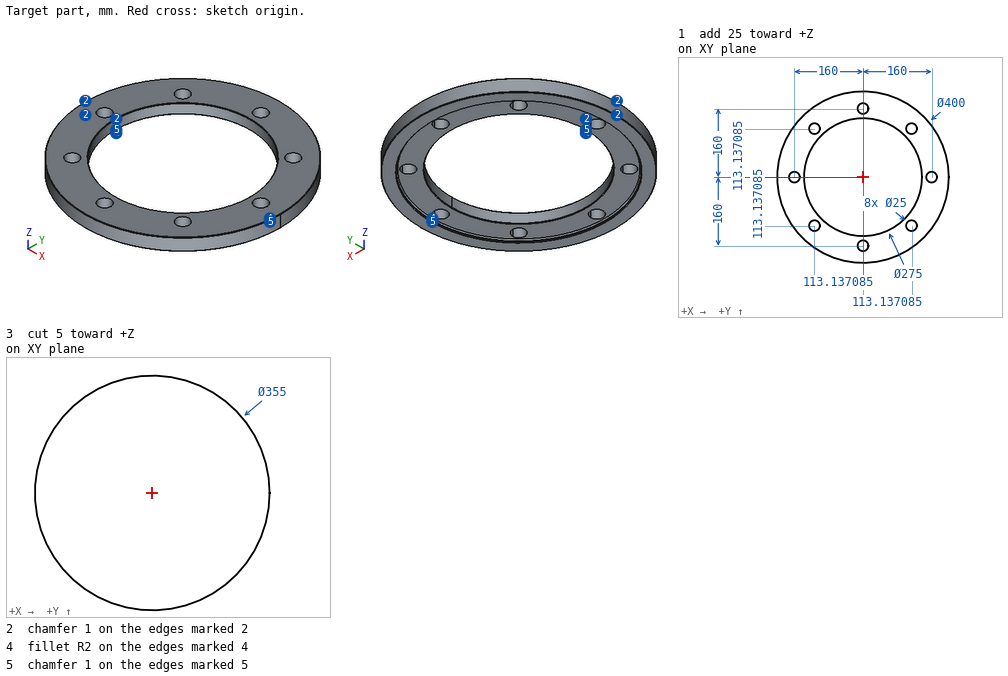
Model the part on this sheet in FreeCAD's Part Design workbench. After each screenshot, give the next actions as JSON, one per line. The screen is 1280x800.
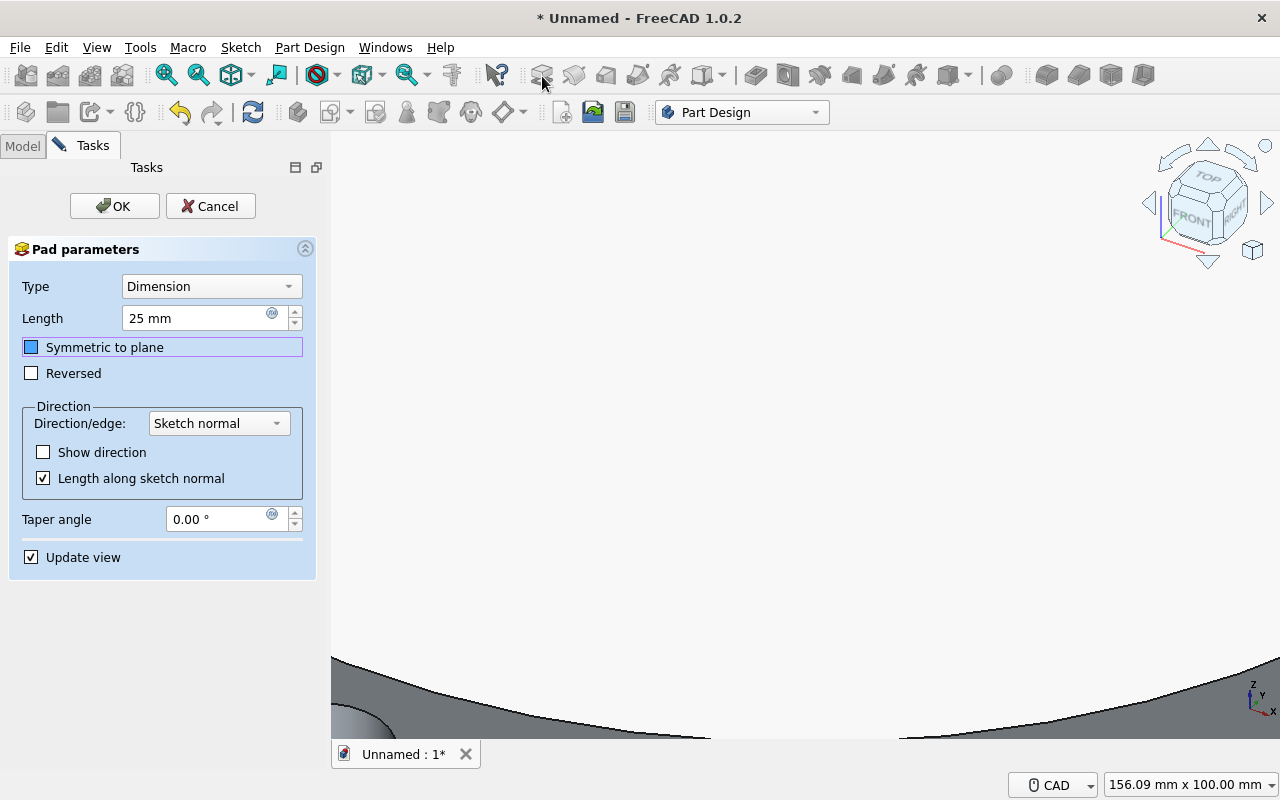
{"action": "left_click", "coordinate": [115, 206]}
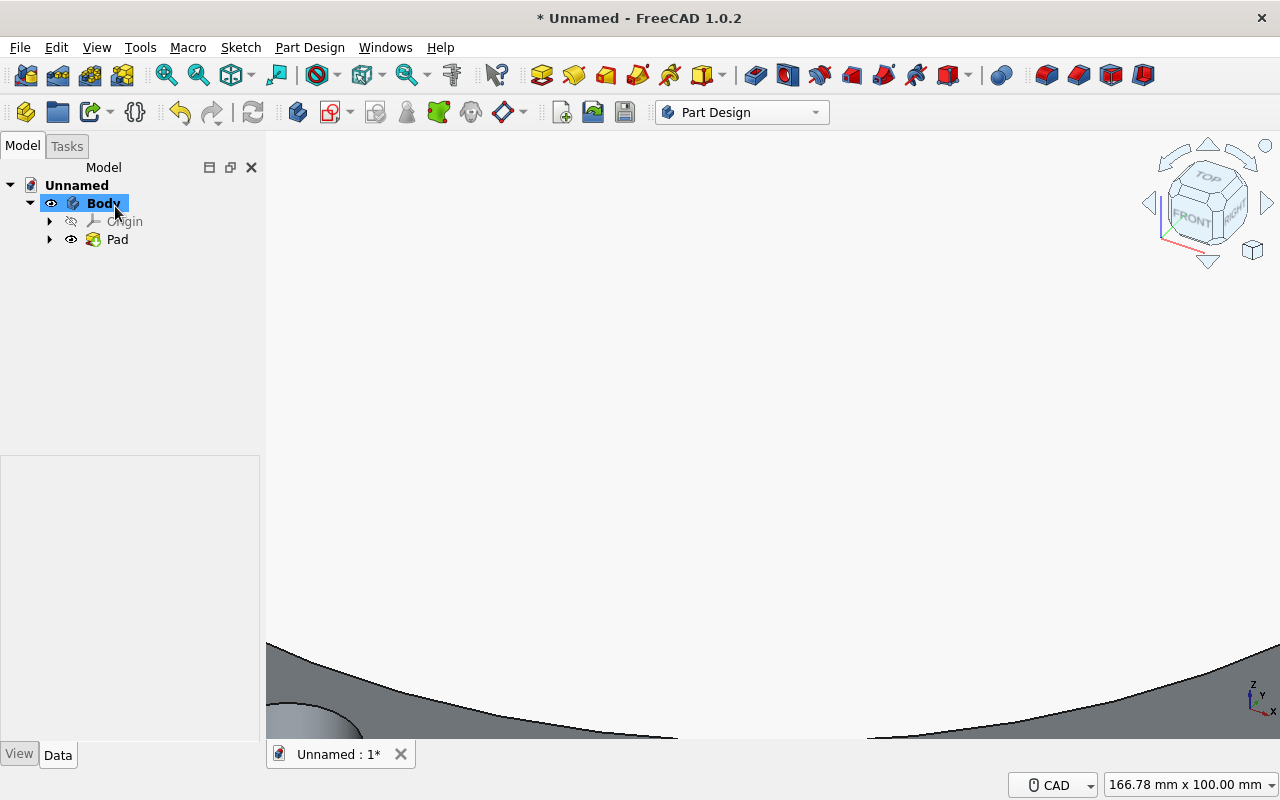
{"action": "left_click", "coordinate": [168, 76]}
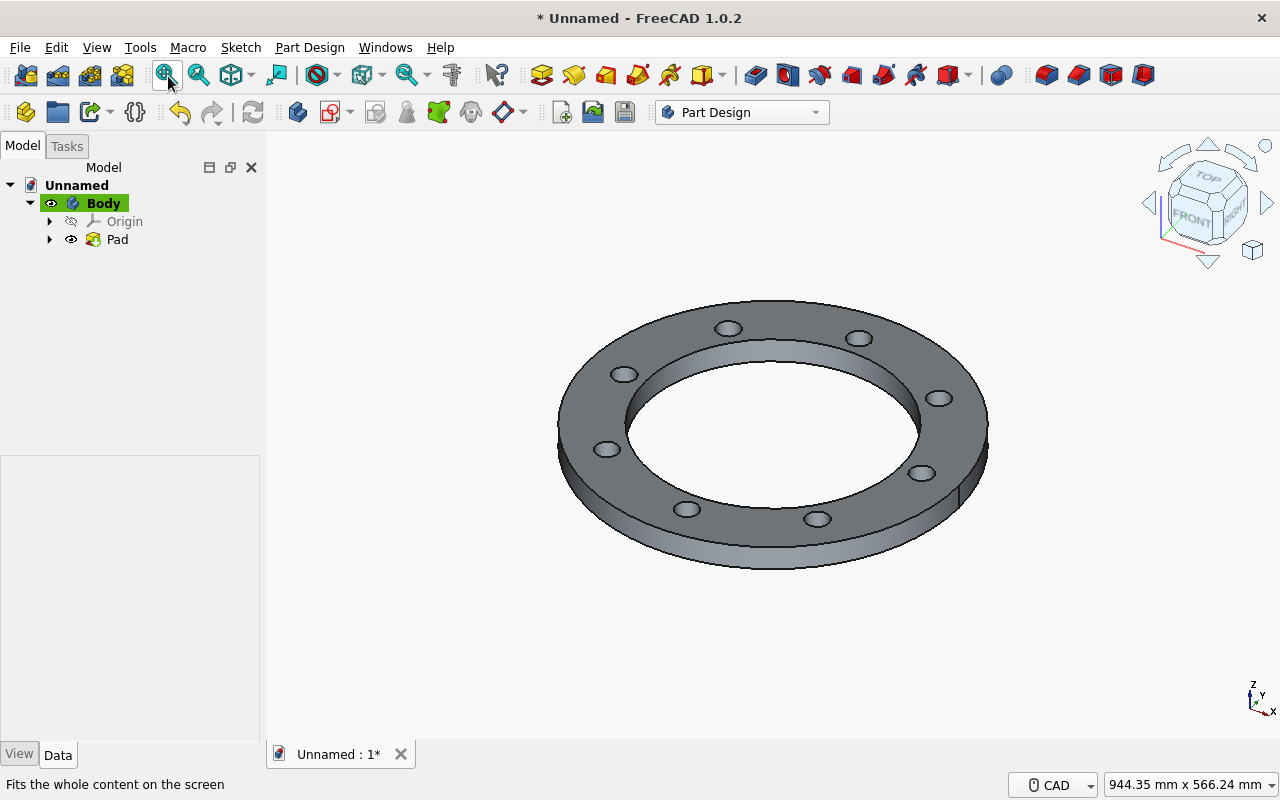
{"action": "left_click", "coordinate": [559, 436]}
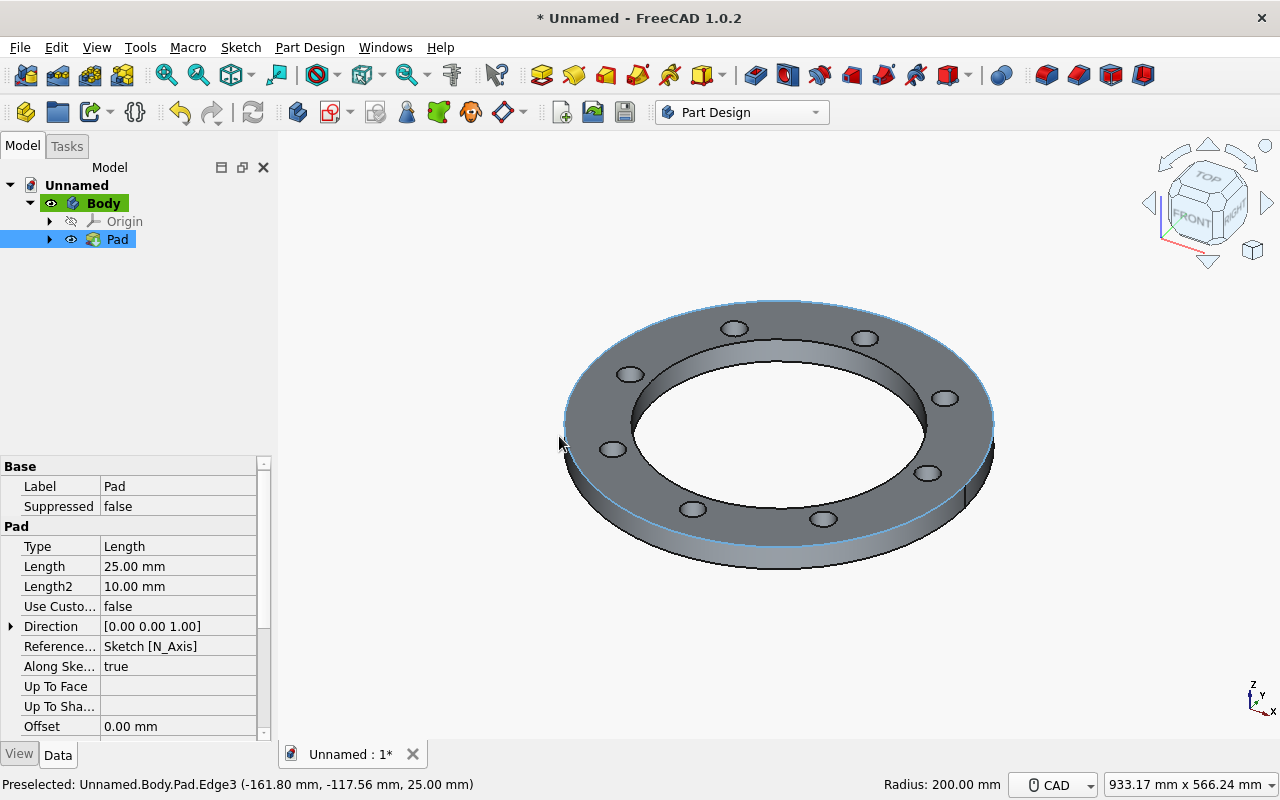
{"action": "left_click", "coordinate": [651, 381], "text": "ctrl"}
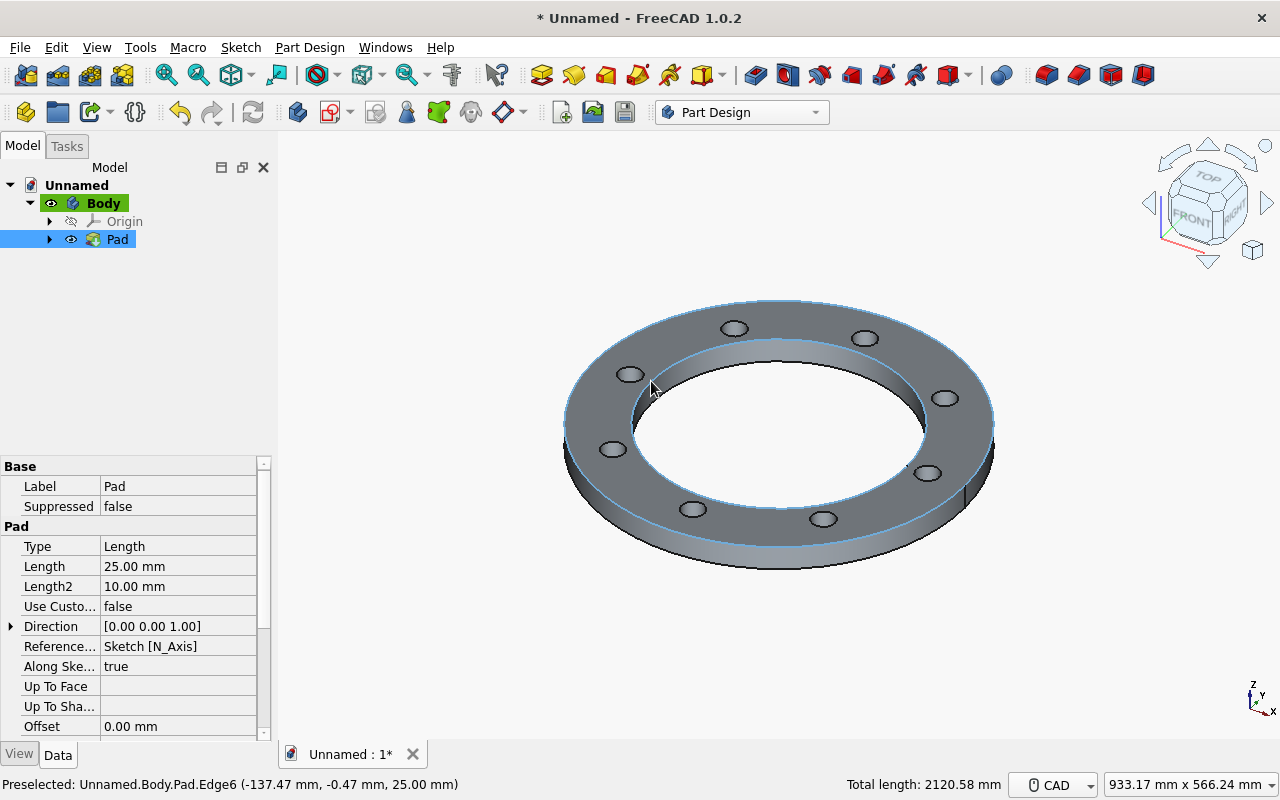
{"action": "key", "text": "0"}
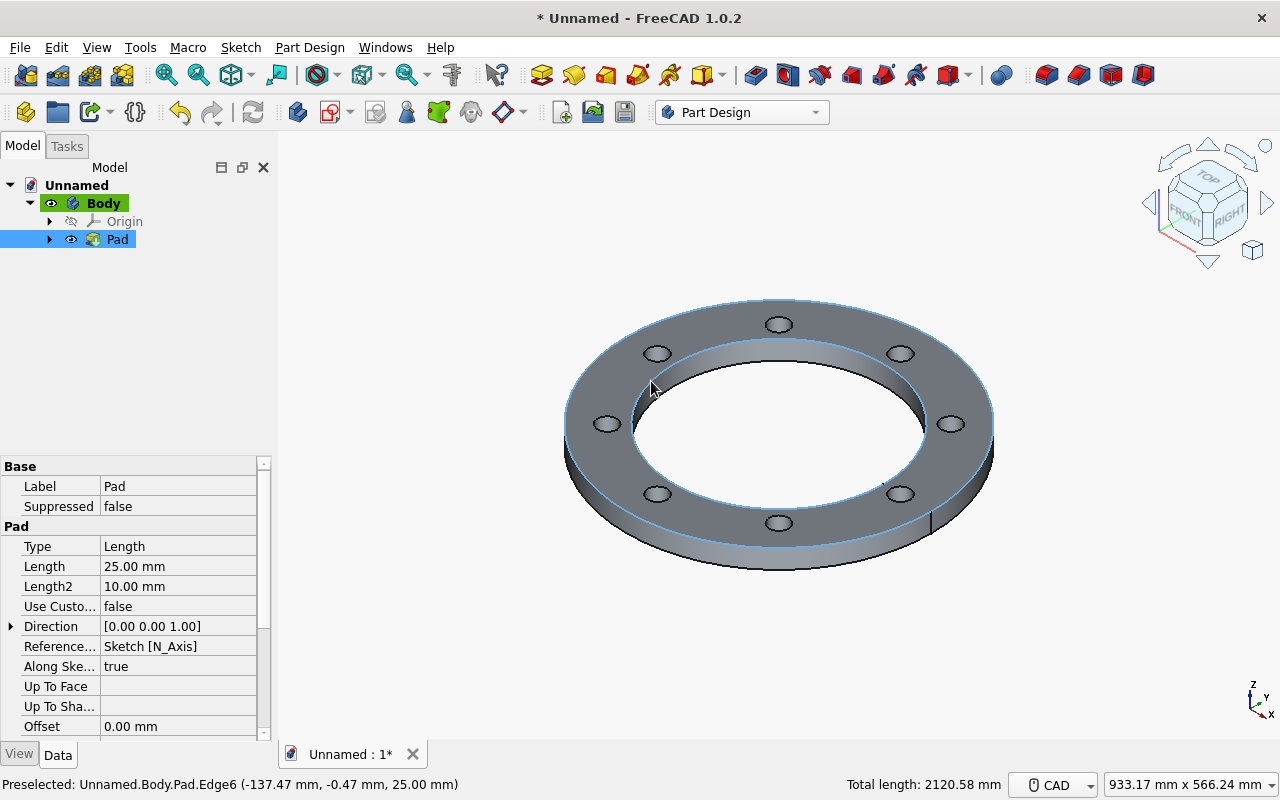
{"action": "key", "text": "2"}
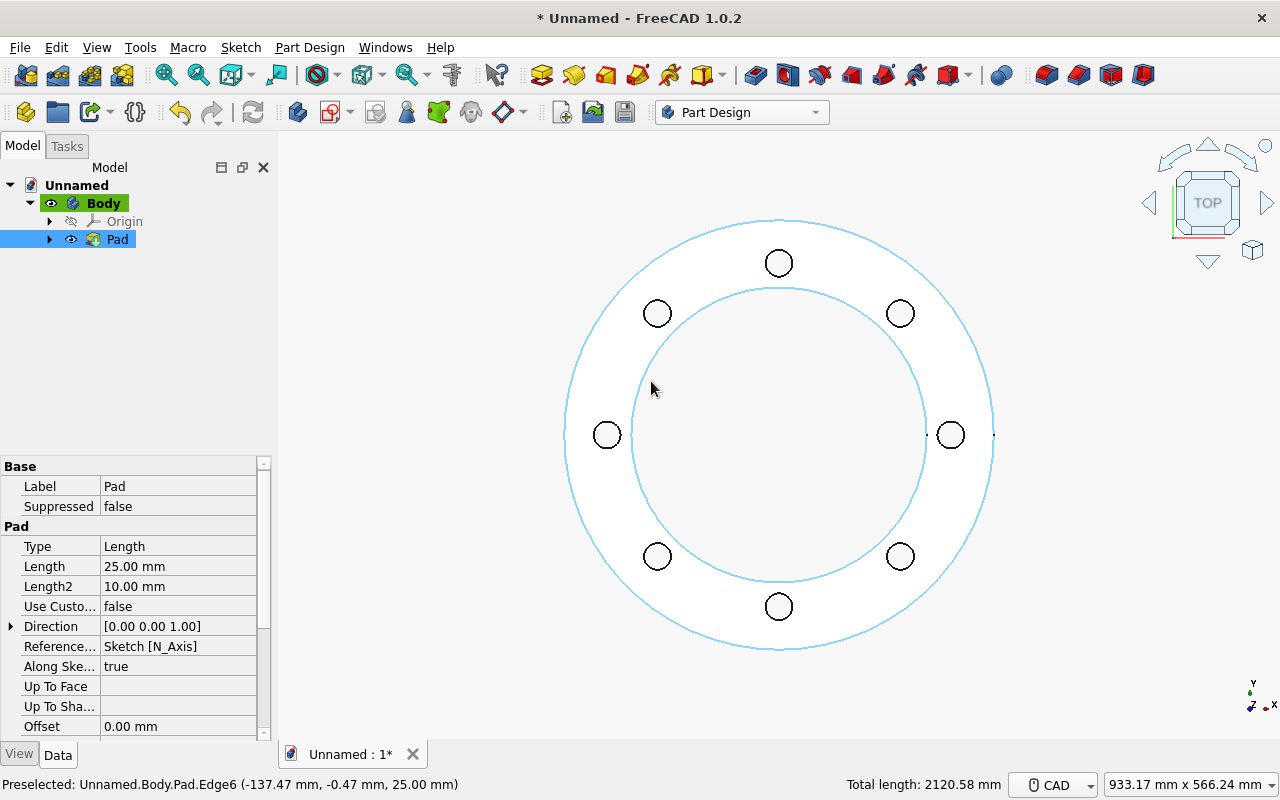
{"action": "key", "text": "1"}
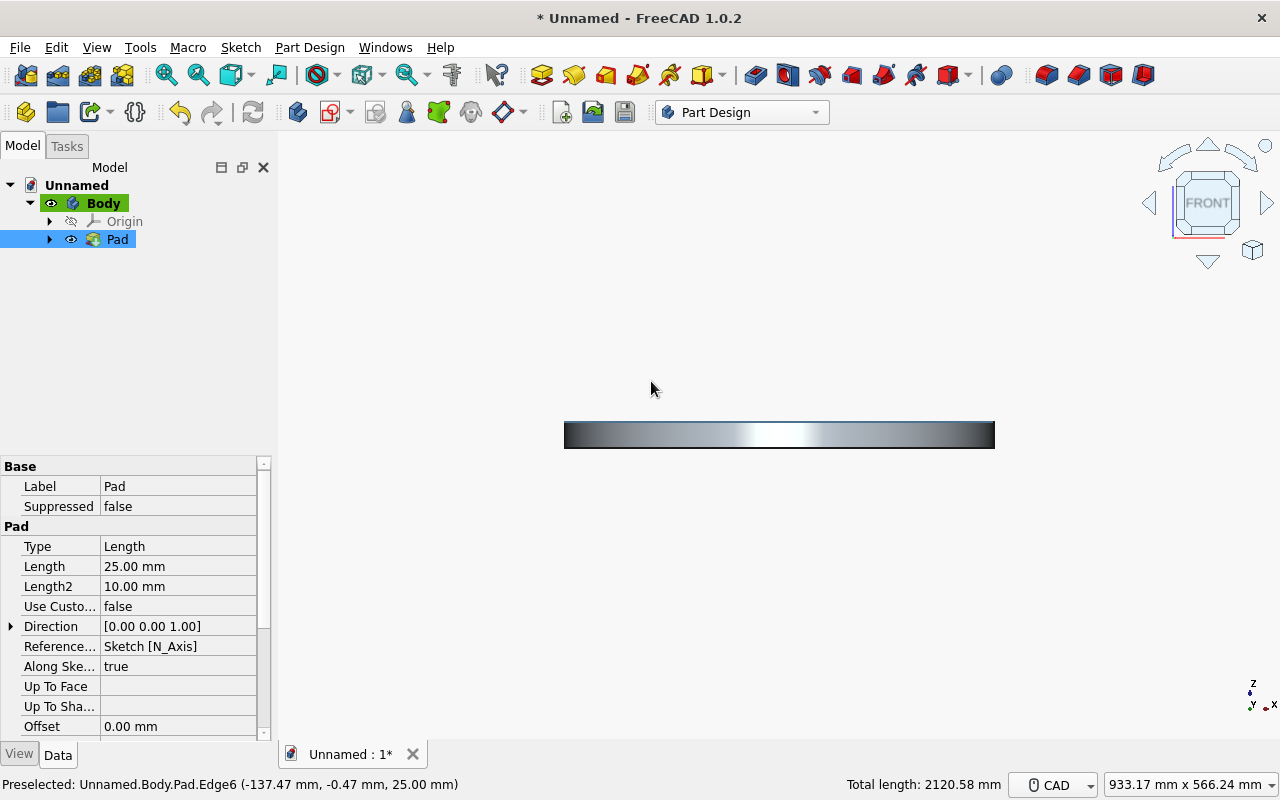
{"action": "left_click", "coordinate": [168, 76]}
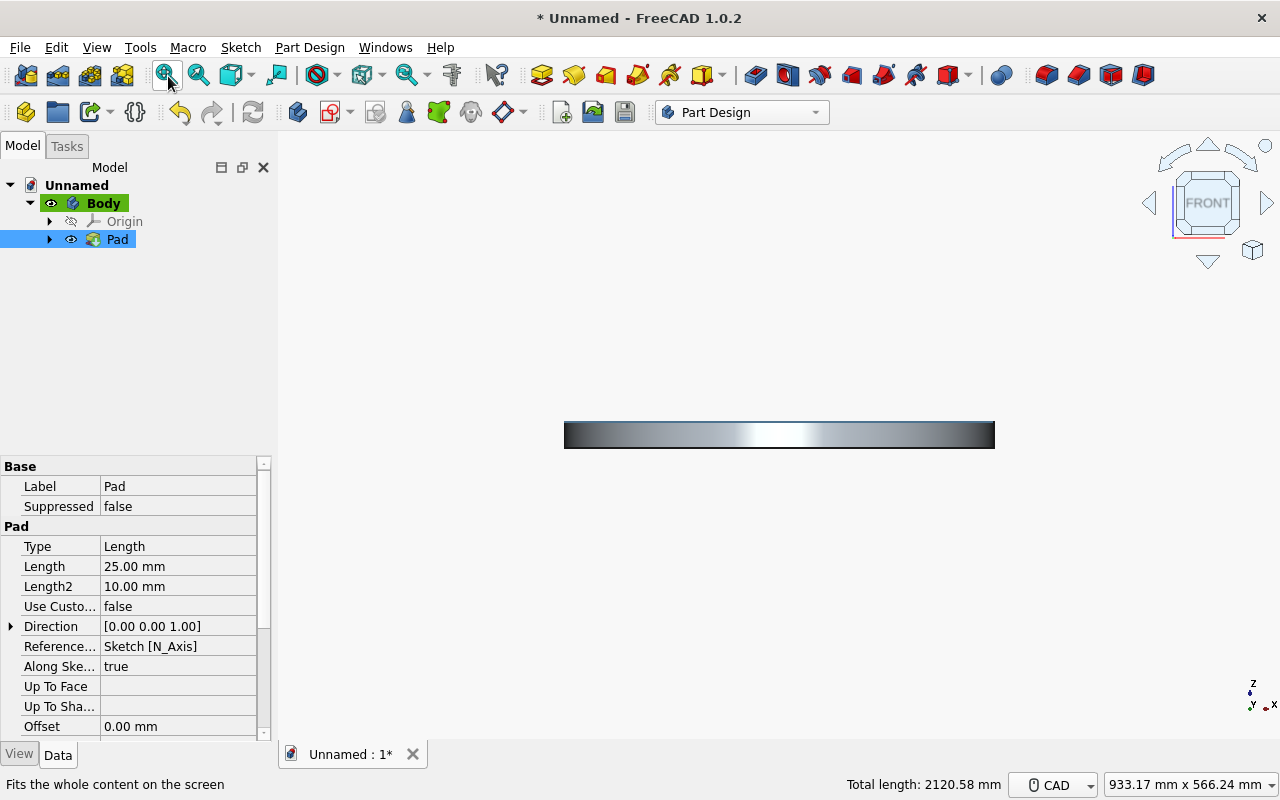
{"action": "left_click", "coordinate": [605, 447], "text": "ctrl"}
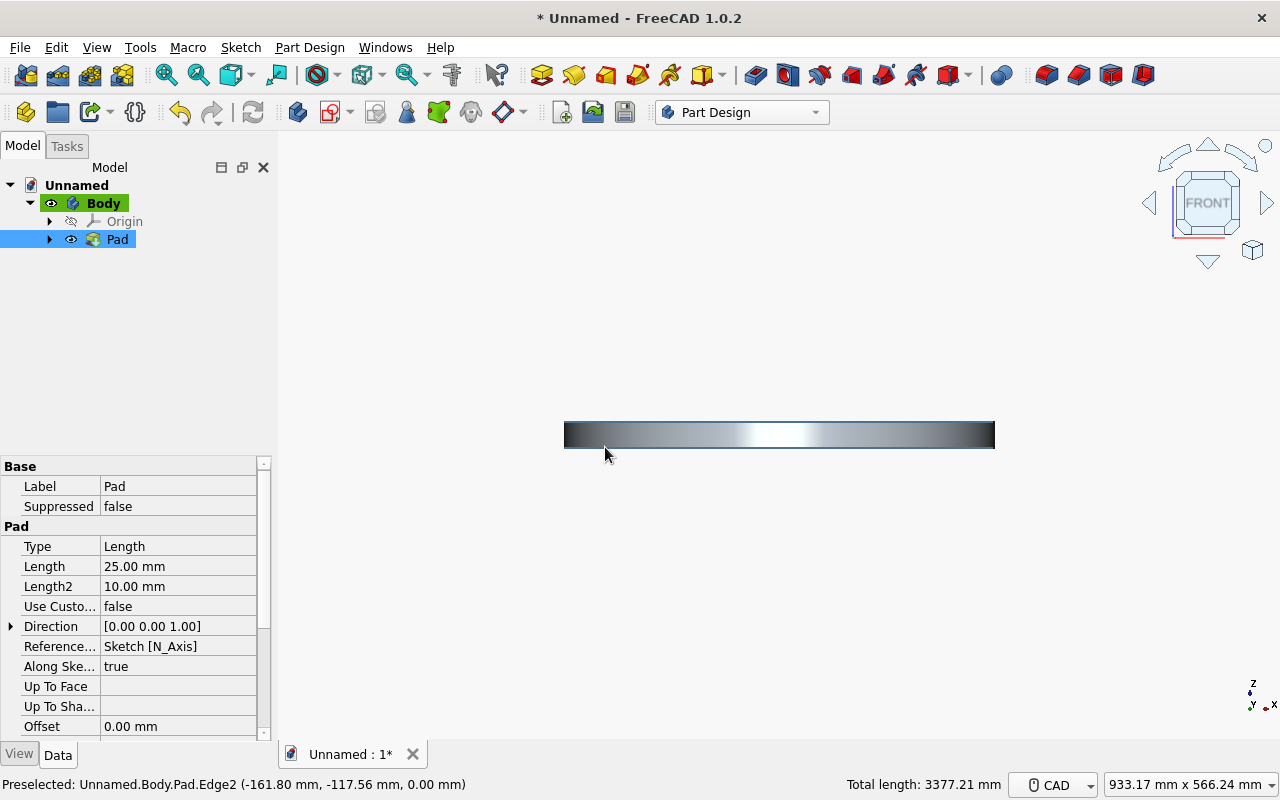
{"action": "key", "text": "3"}